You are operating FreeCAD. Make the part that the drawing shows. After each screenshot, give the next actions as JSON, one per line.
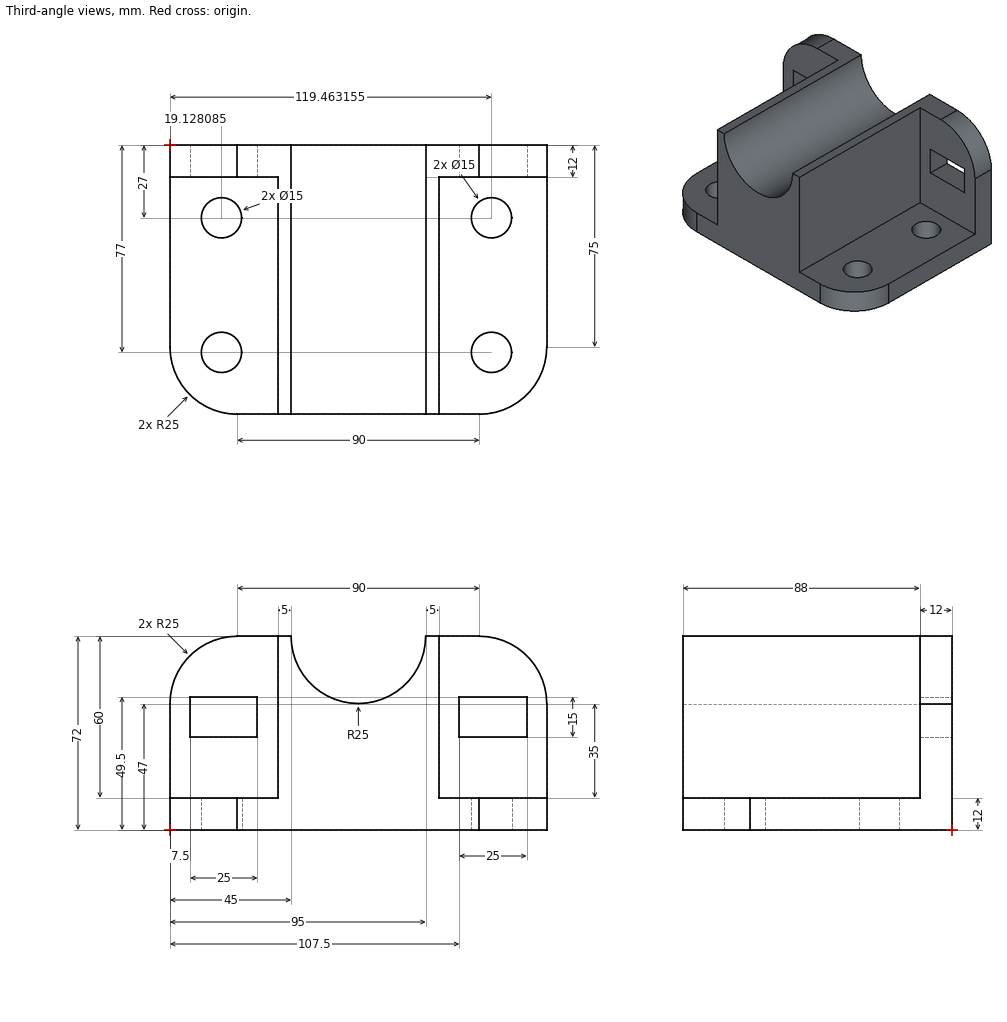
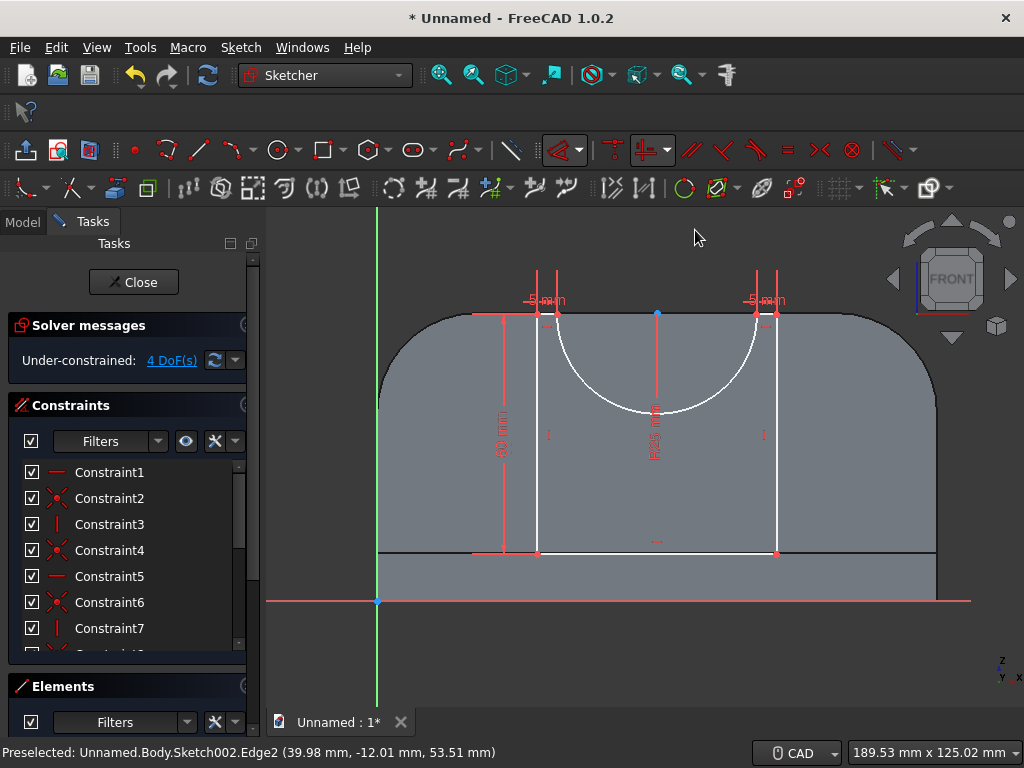
{"action": "left_click", "coordinate": [777, 482]}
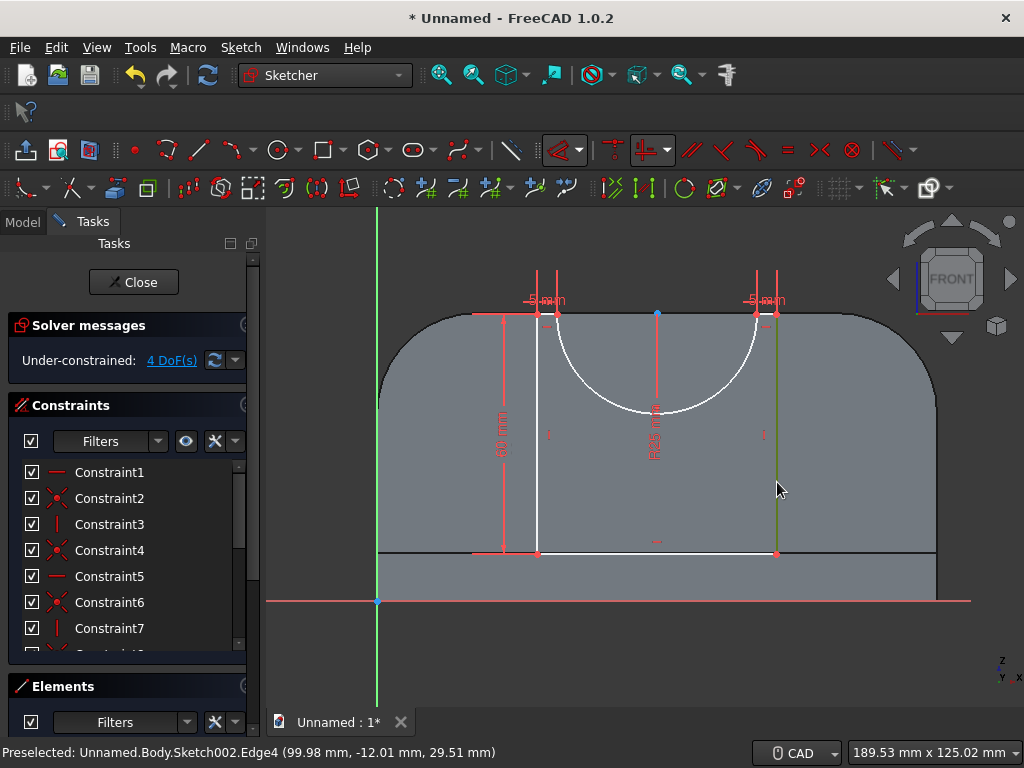
{"action": "key", "text": "i"}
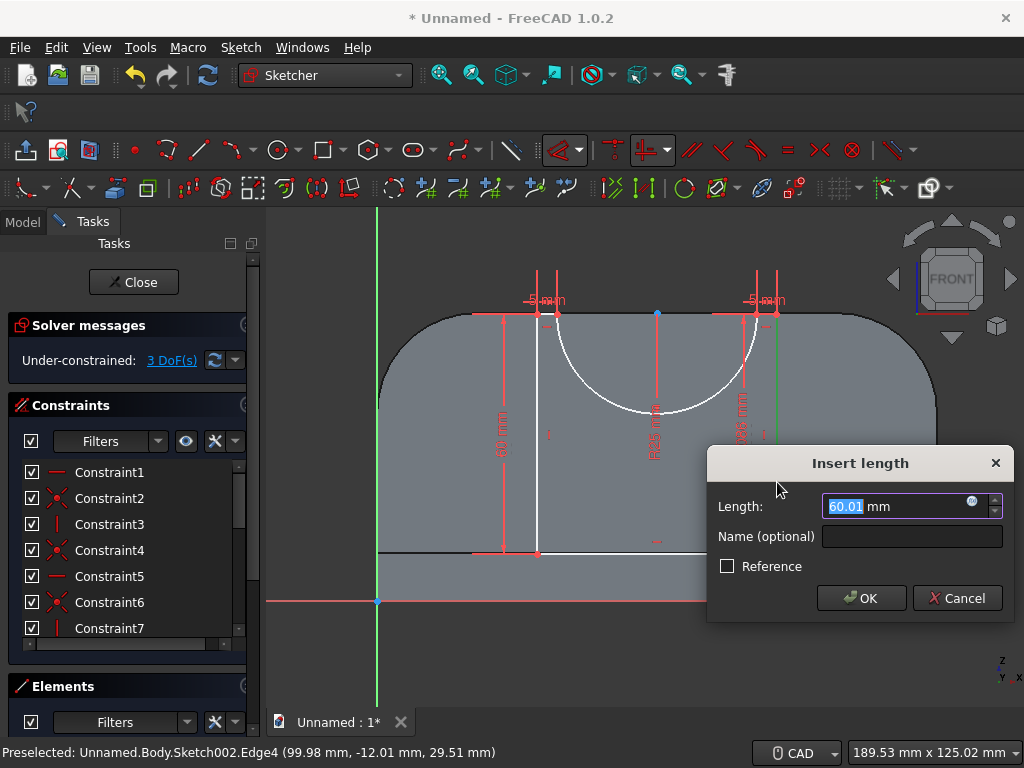
{"action": "type", "text": "60"}
{"action": "key", "text": "Return"}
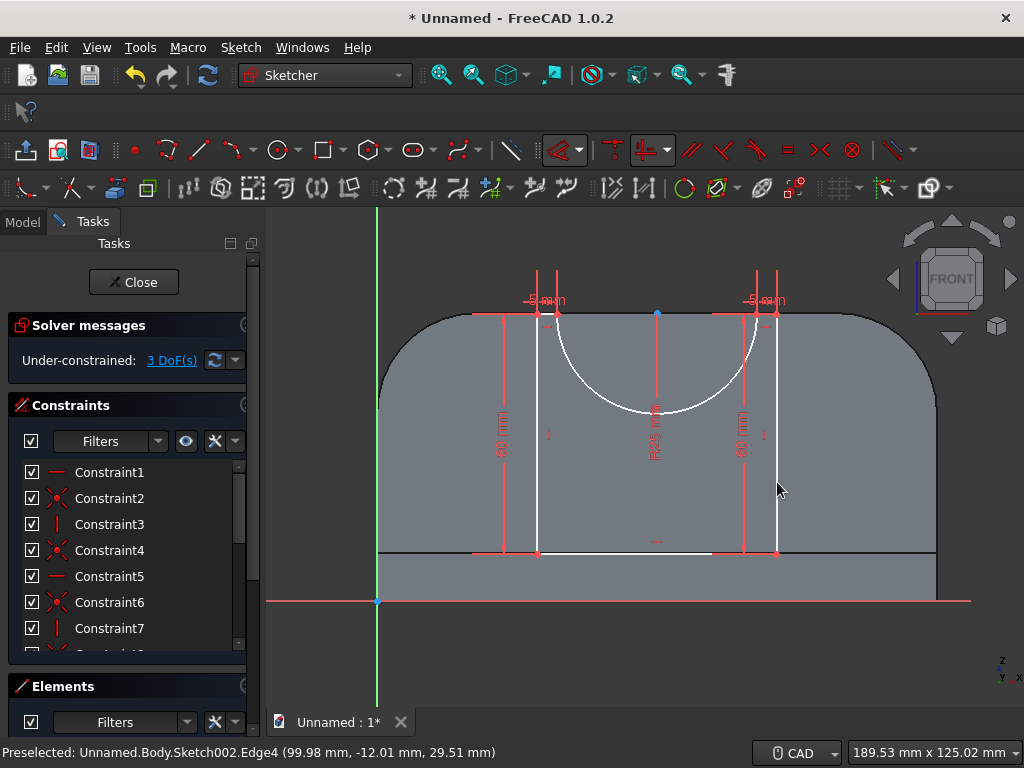
{"action": "left_click", "coordinate": [557, 314]}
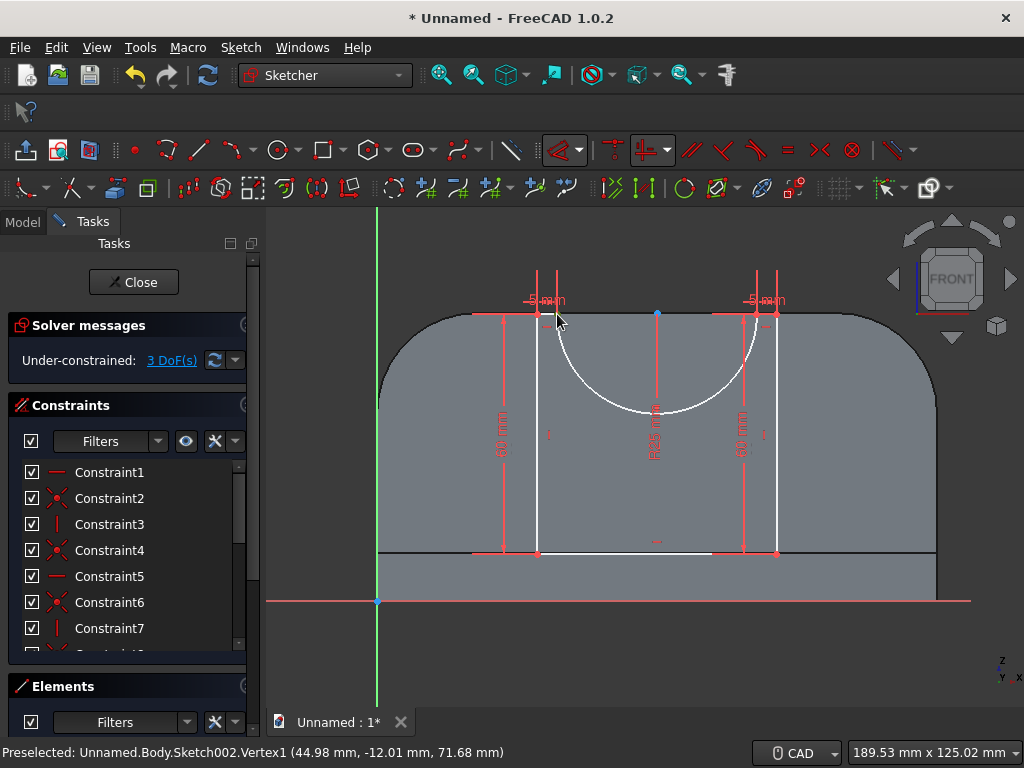
{"action": "key", "text": "l"}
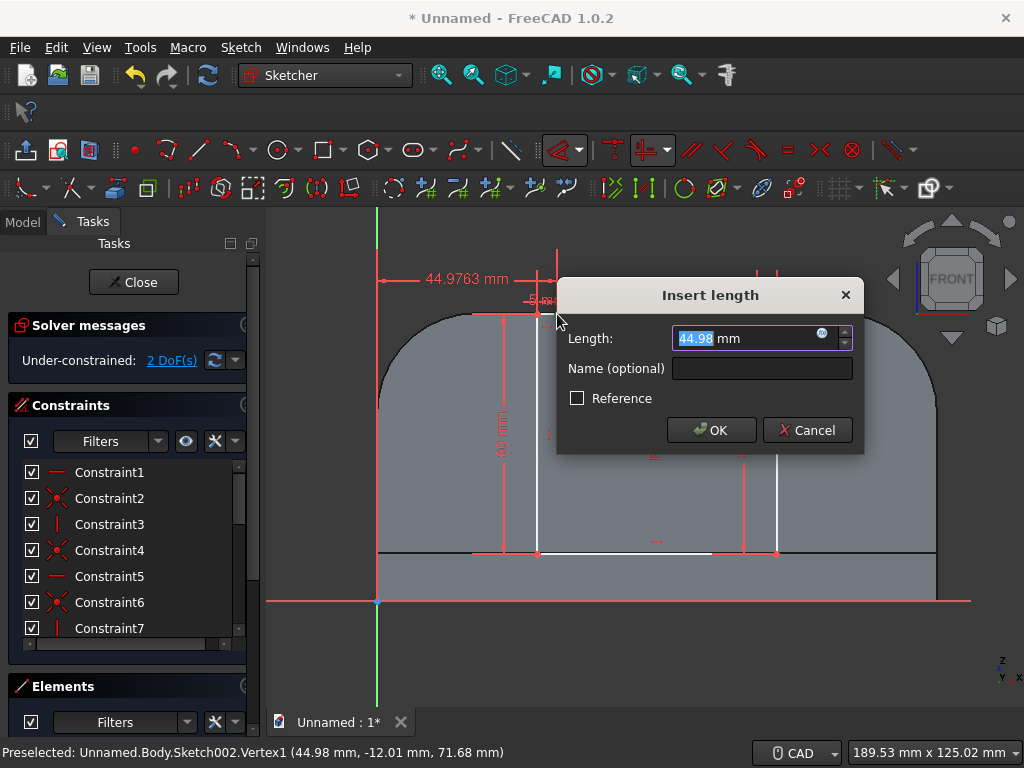
{"action": "type", "text": "45"}
{"action": "key", "text": "Return"}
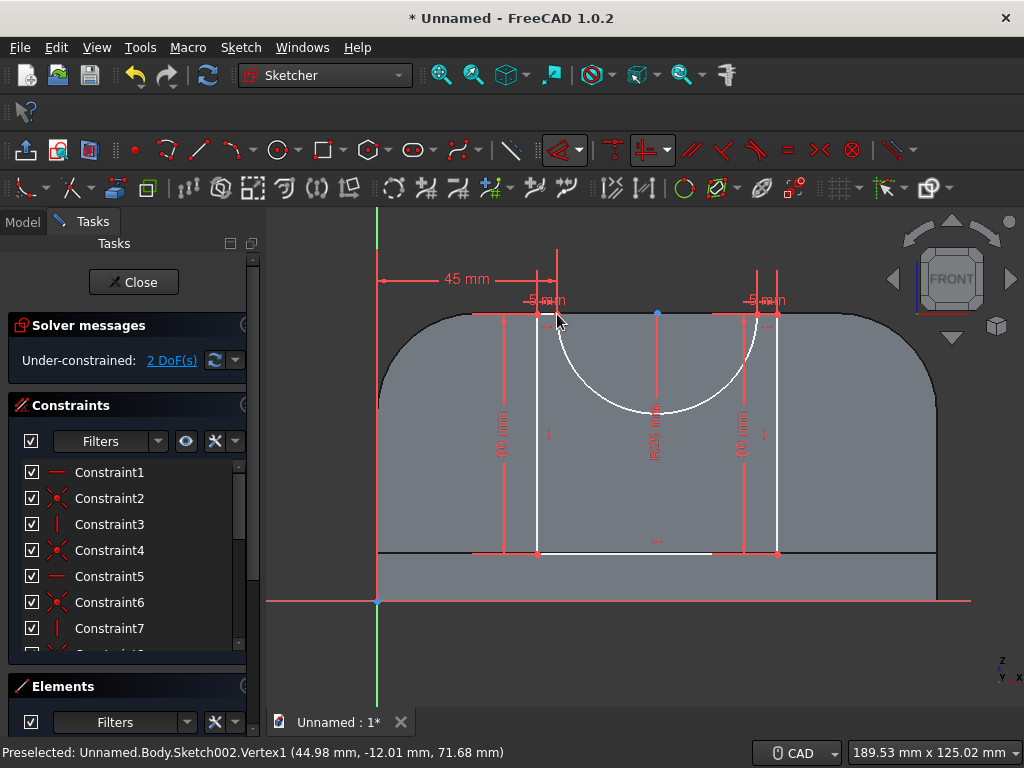
{"action": "left_click", "coordinate": [557, 314]}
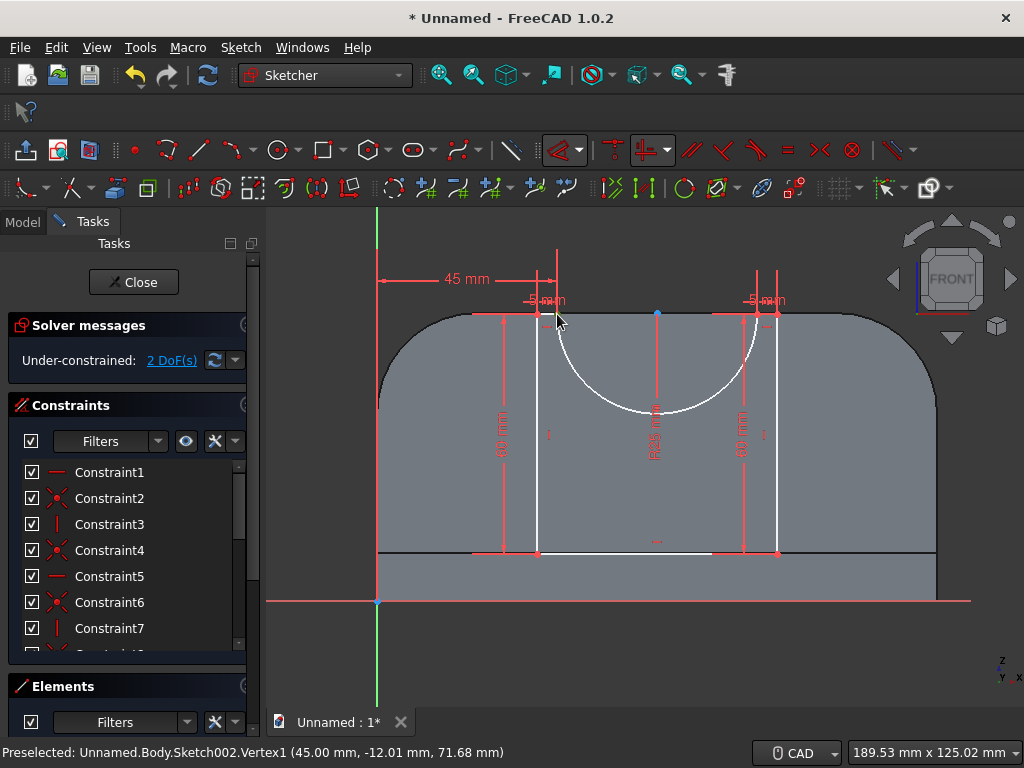
{"action": "key", "text": "i"}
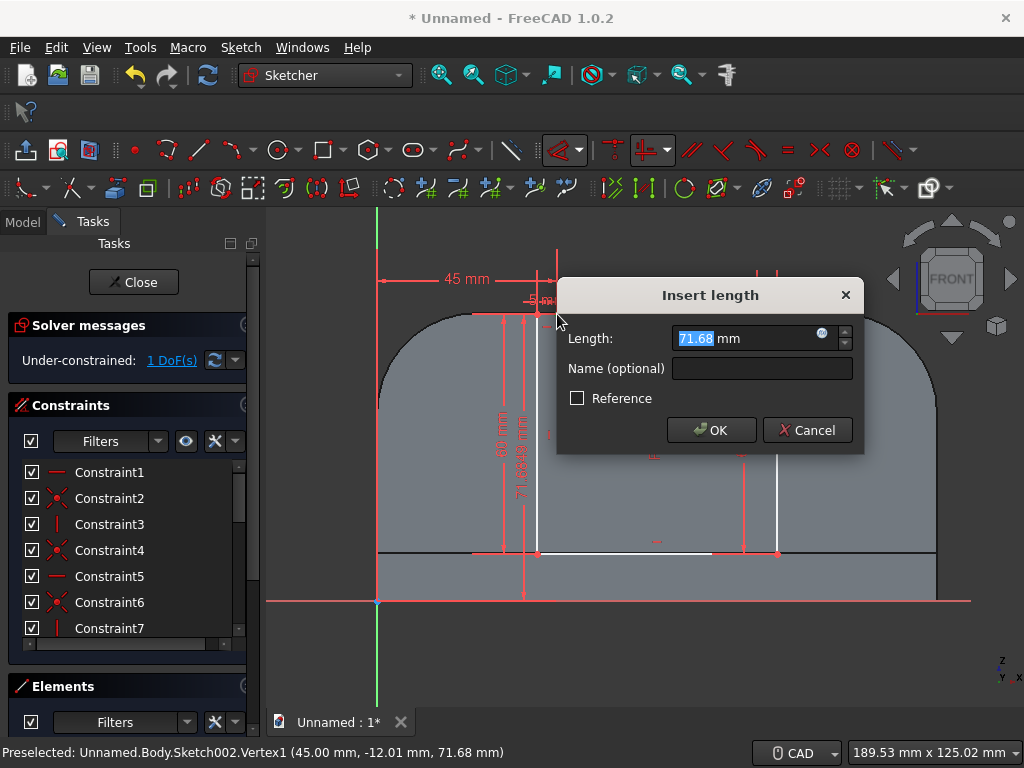
{"action": "type", "text": "72"}
{"action": "key", "text": "Return"}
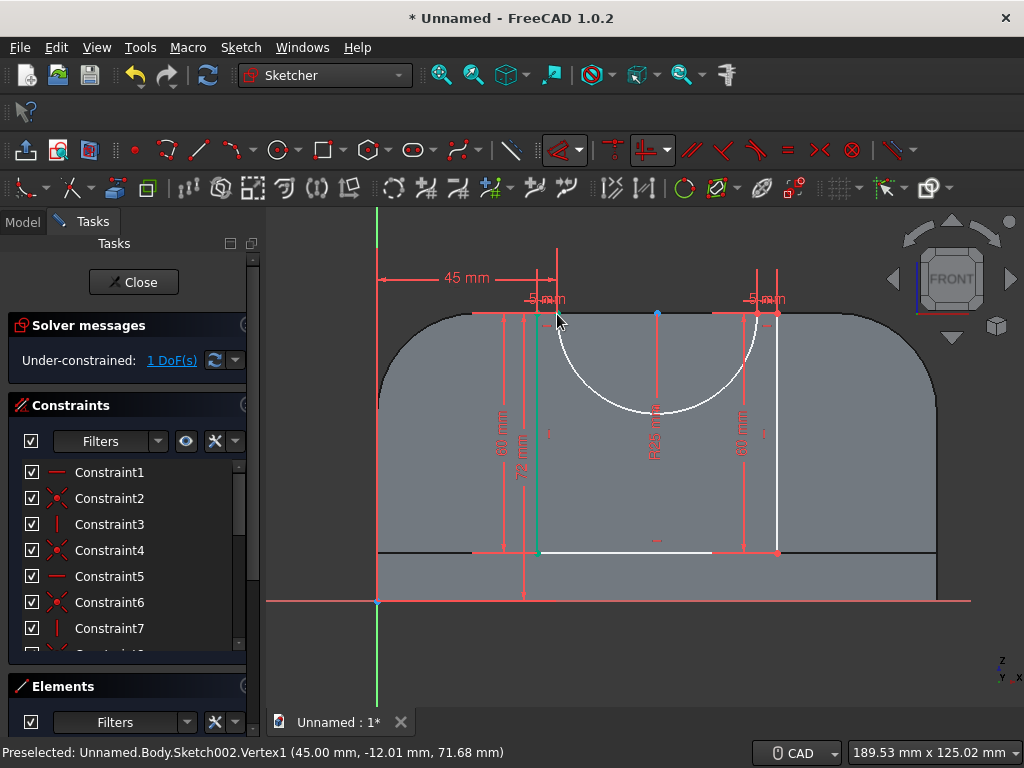
{"action": "left_click", "coordinate": [657, 314]}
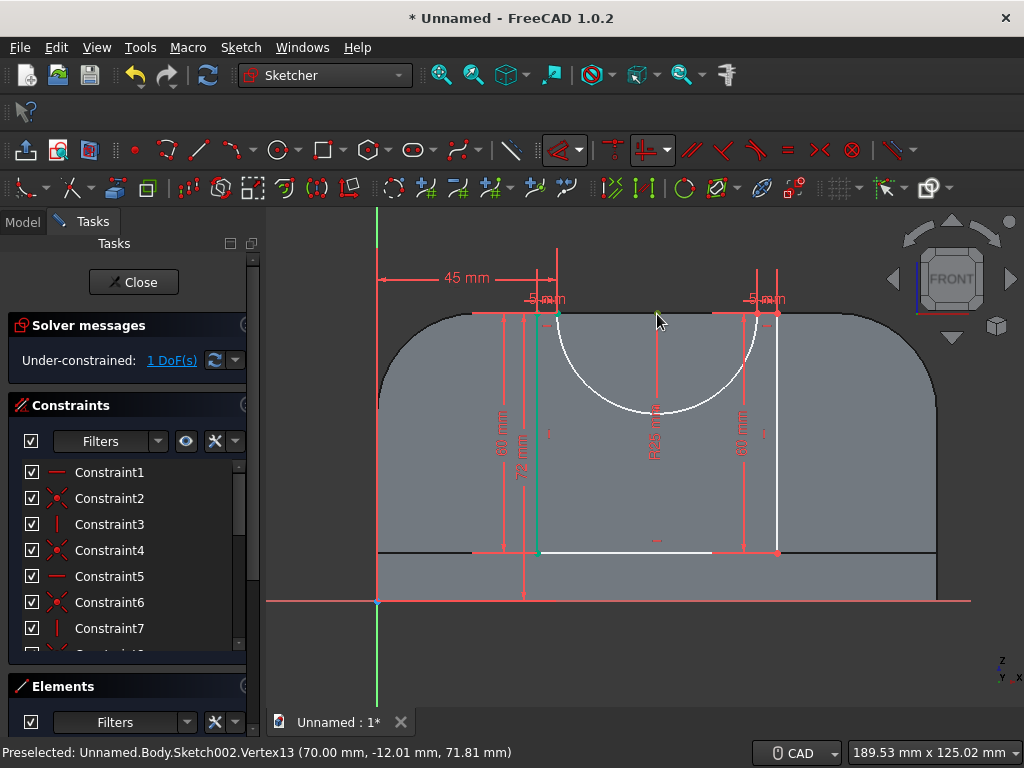
{"action": "key", "text": "i"}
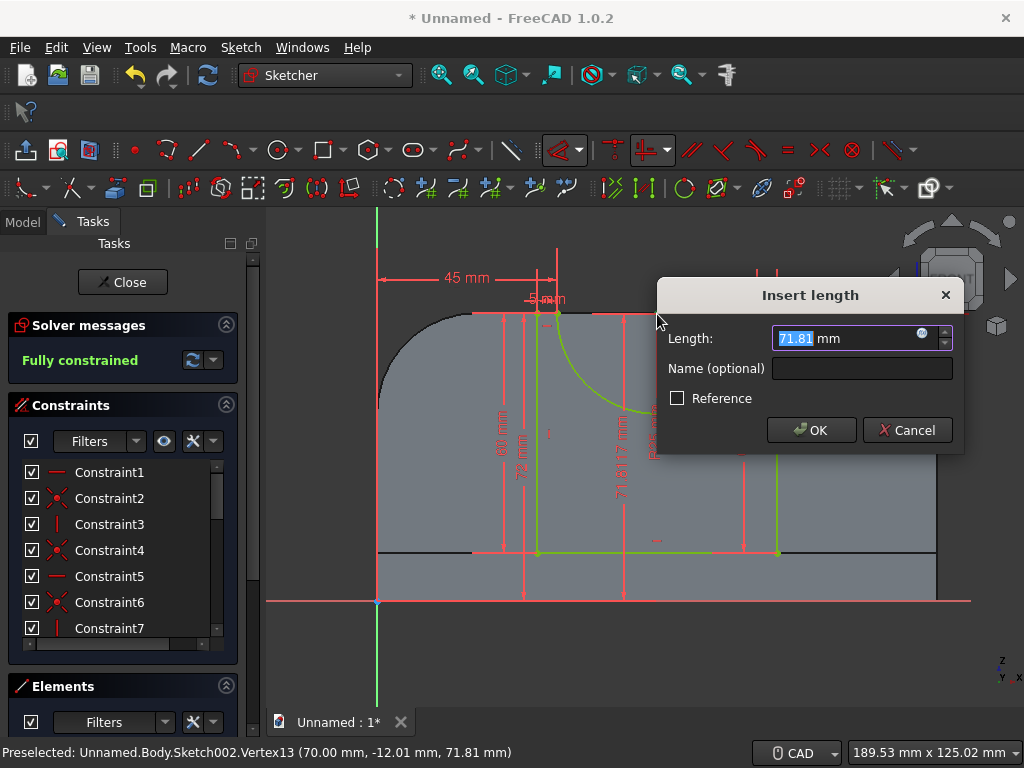
{"action": "type", "text": "72"}
{"action": "key", "text": "Return"}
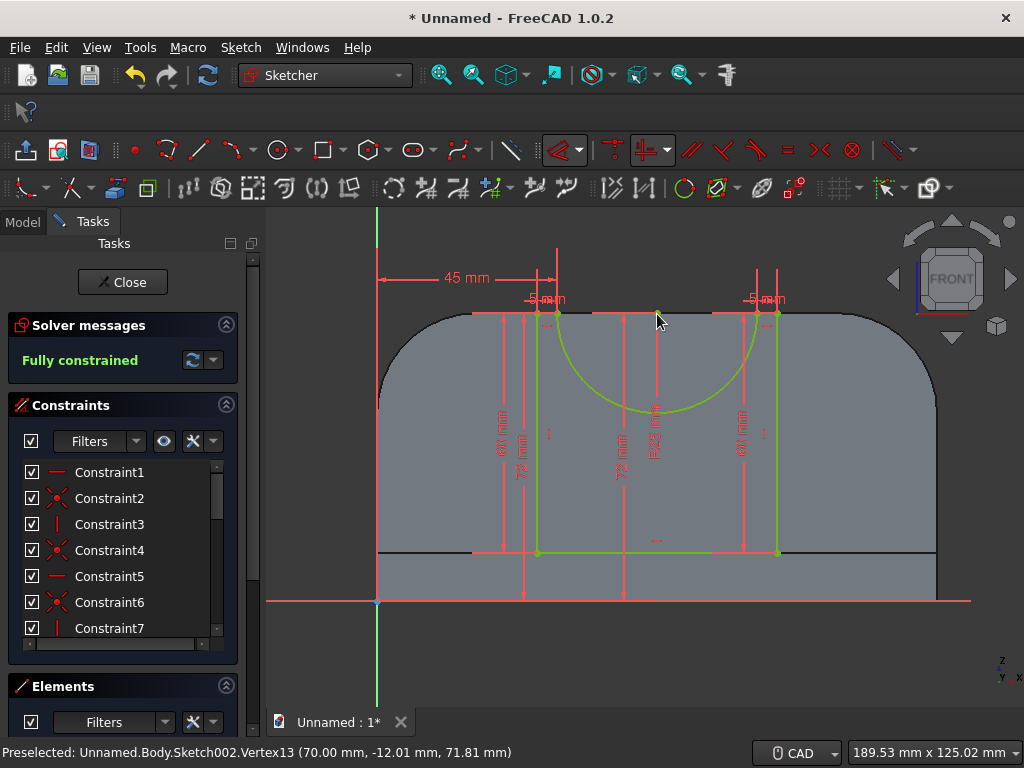
{"action": "left_click", "coordinate": [123, 282]}